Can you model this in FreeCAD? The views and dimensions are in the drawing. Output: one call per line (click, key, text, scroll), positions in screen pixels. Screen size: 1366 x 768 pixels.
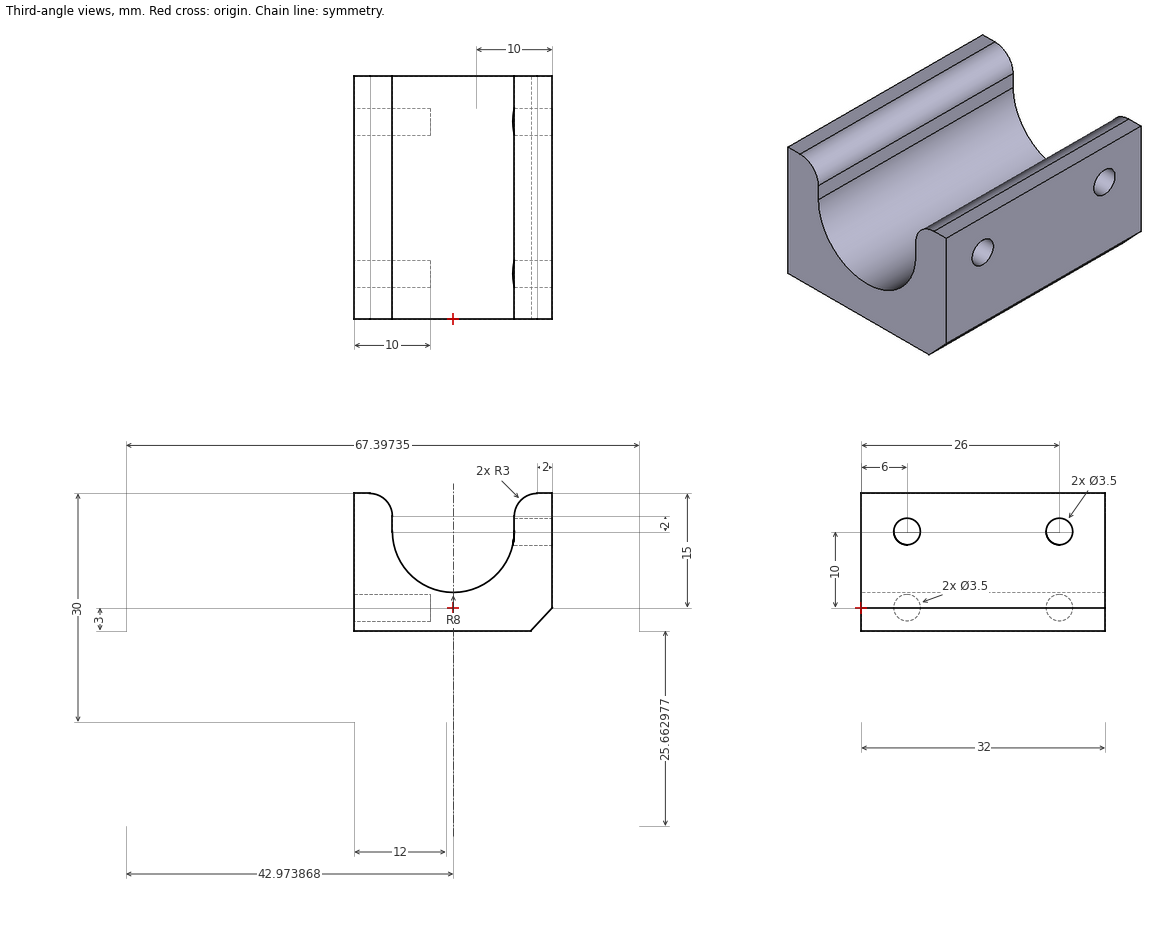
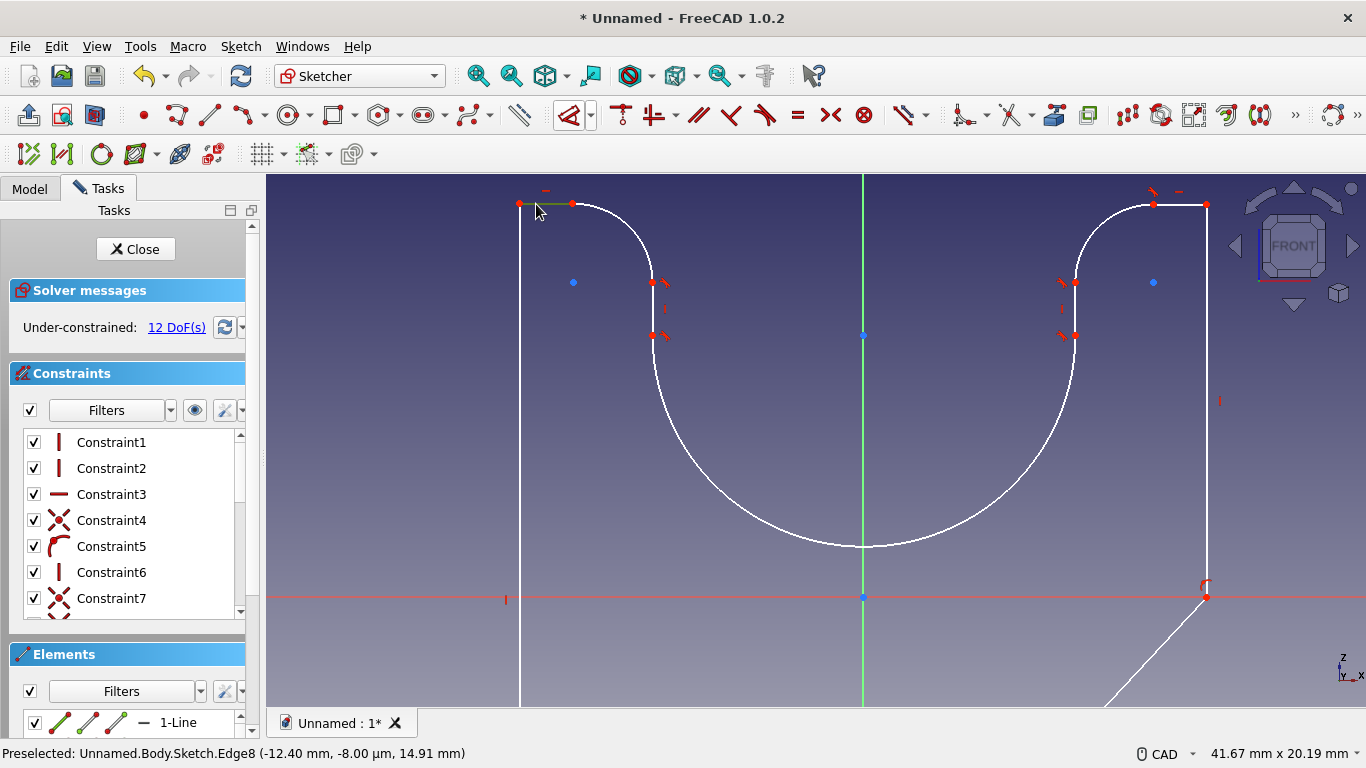
click(644, 246)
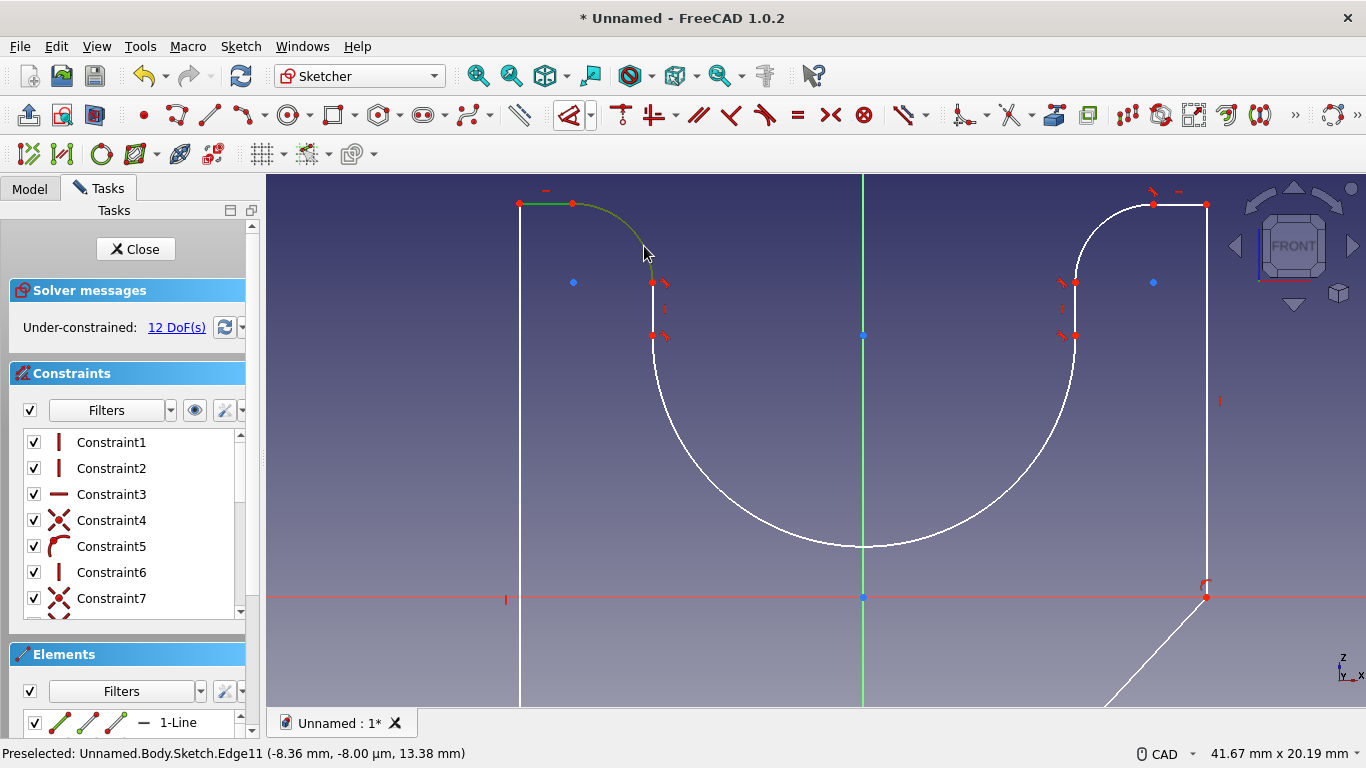
click(765, 116)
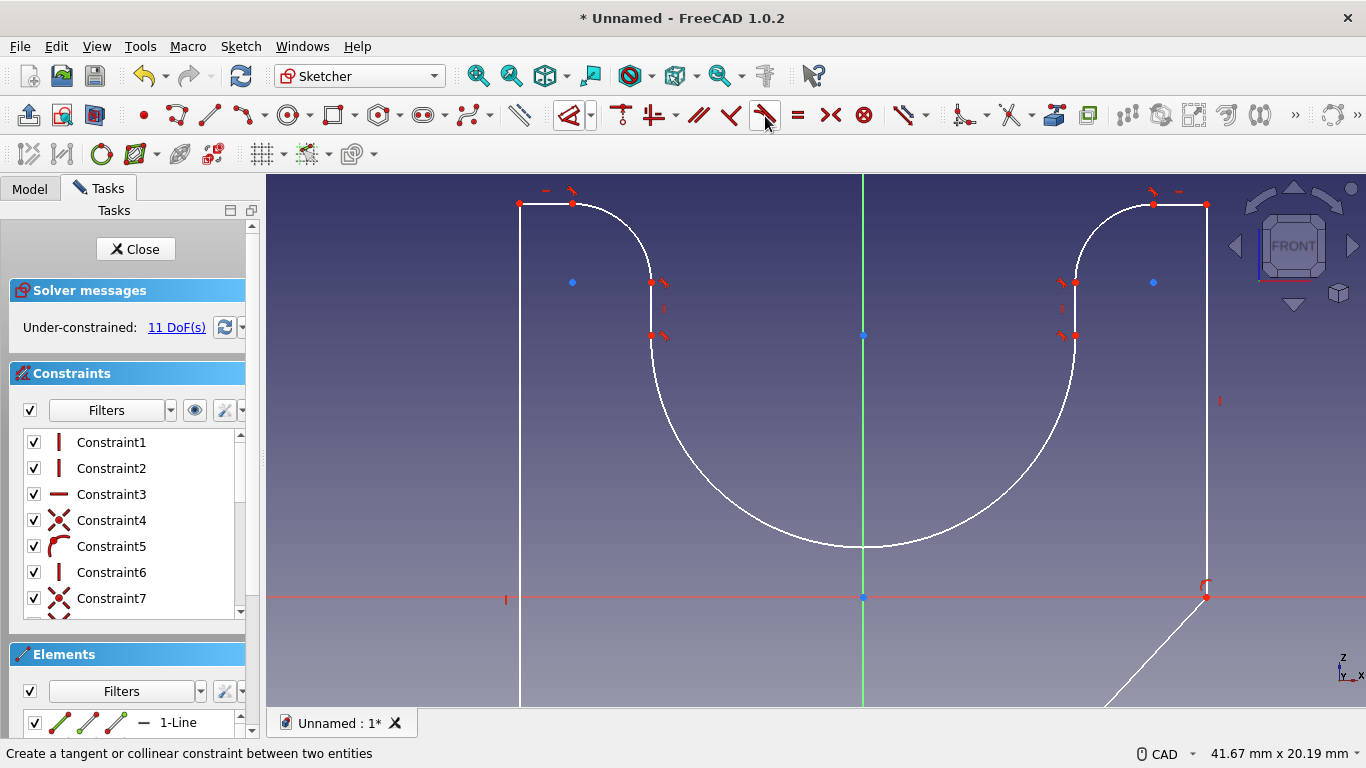
click(1118, 213)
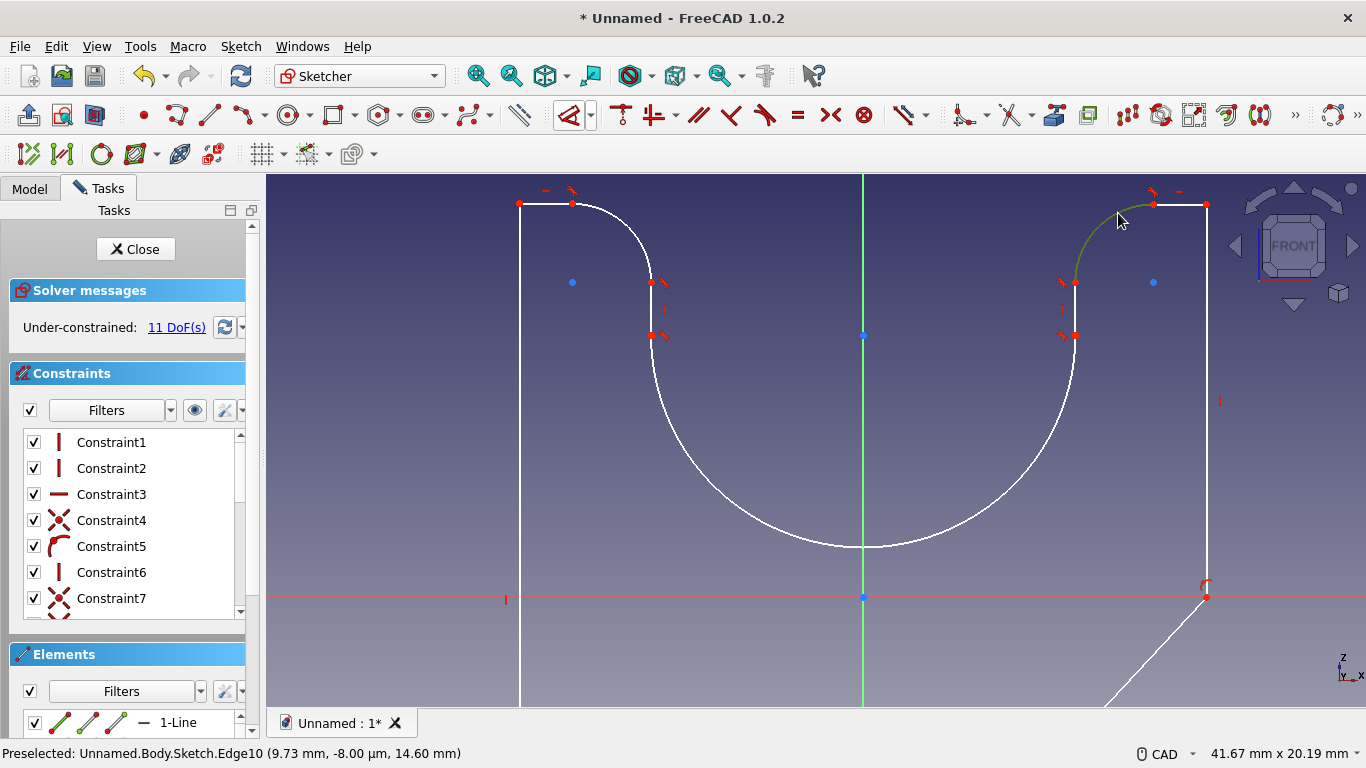
click(642, 247)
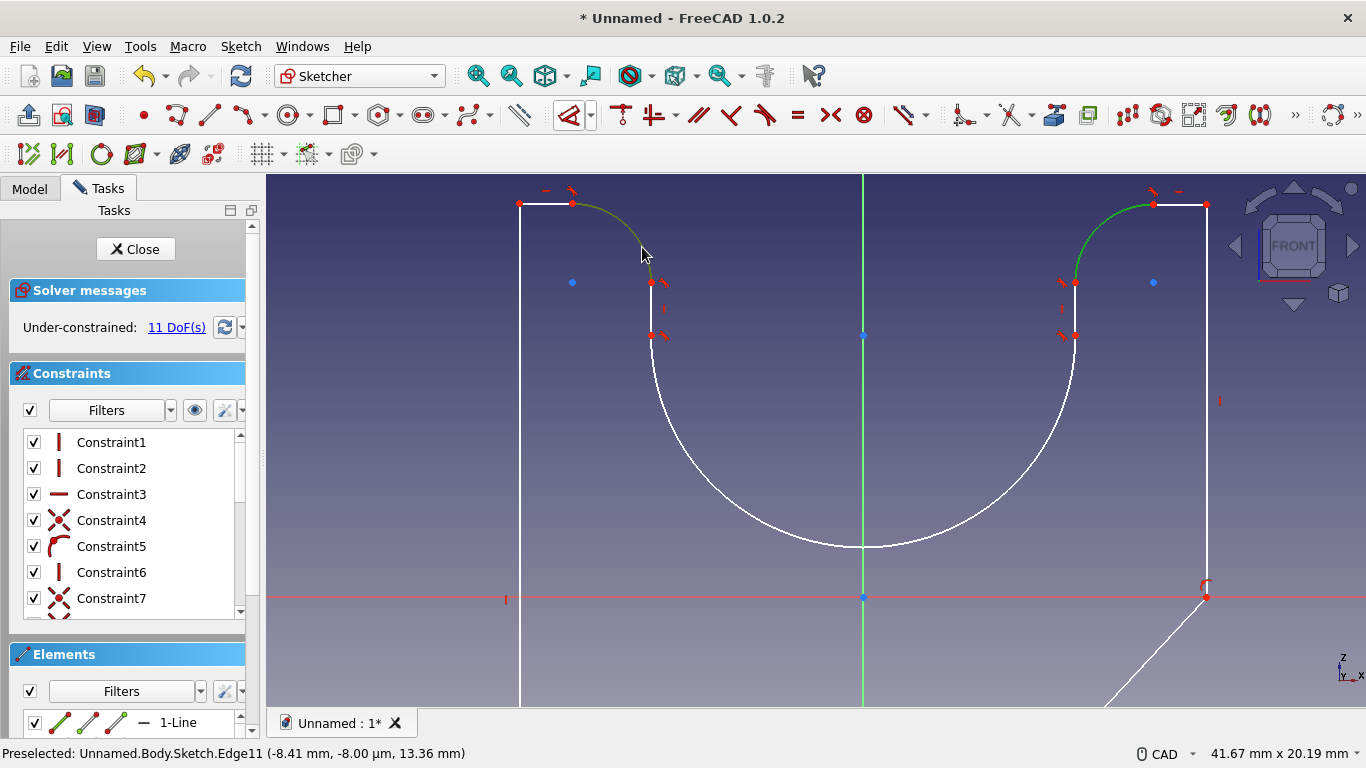
click(798, 116)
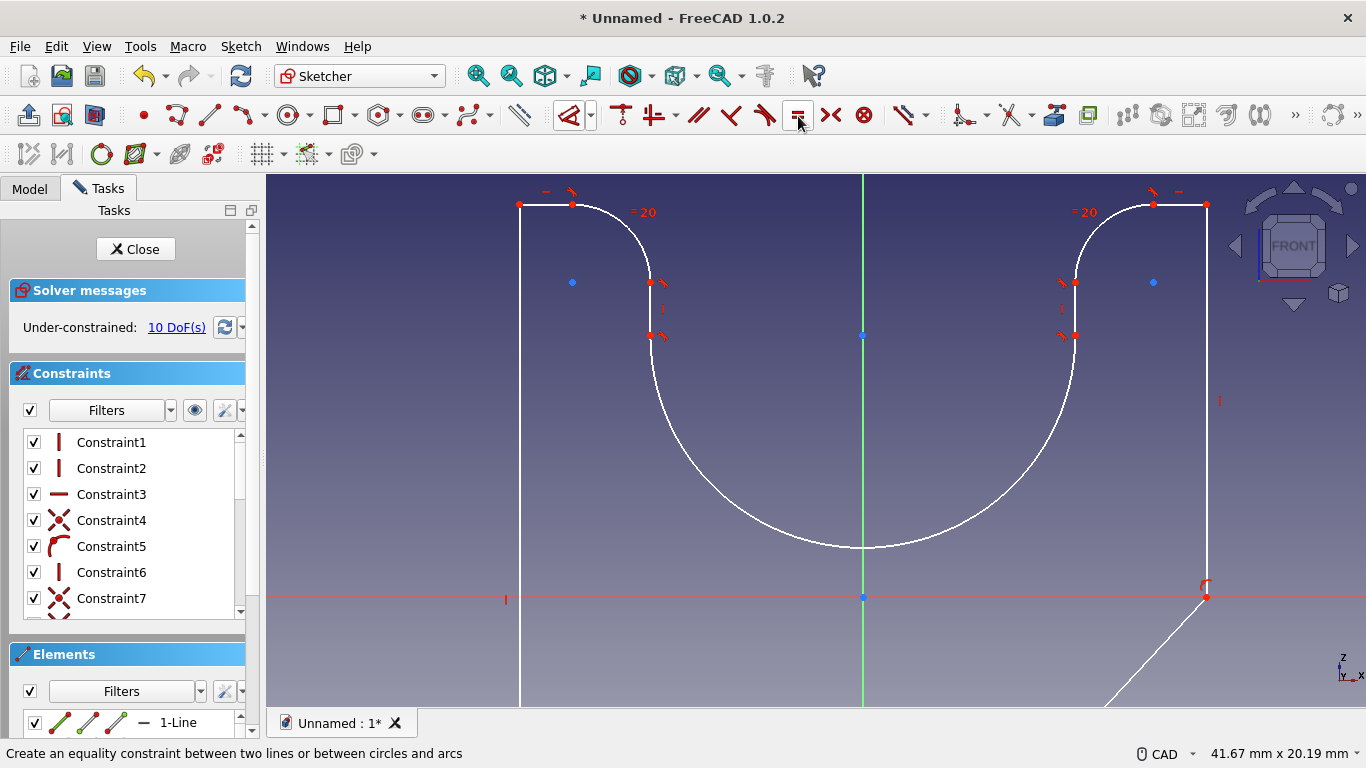
click(863, 335)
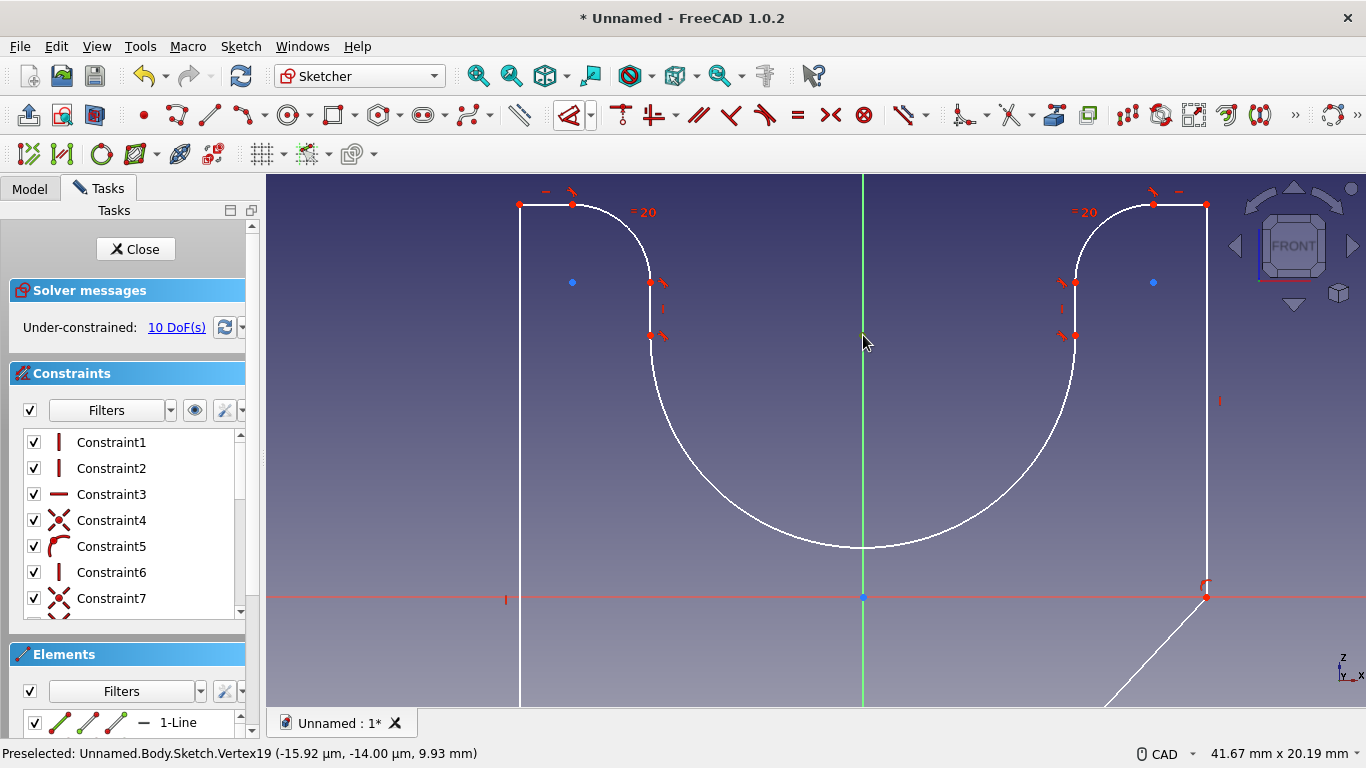
click(863, 645)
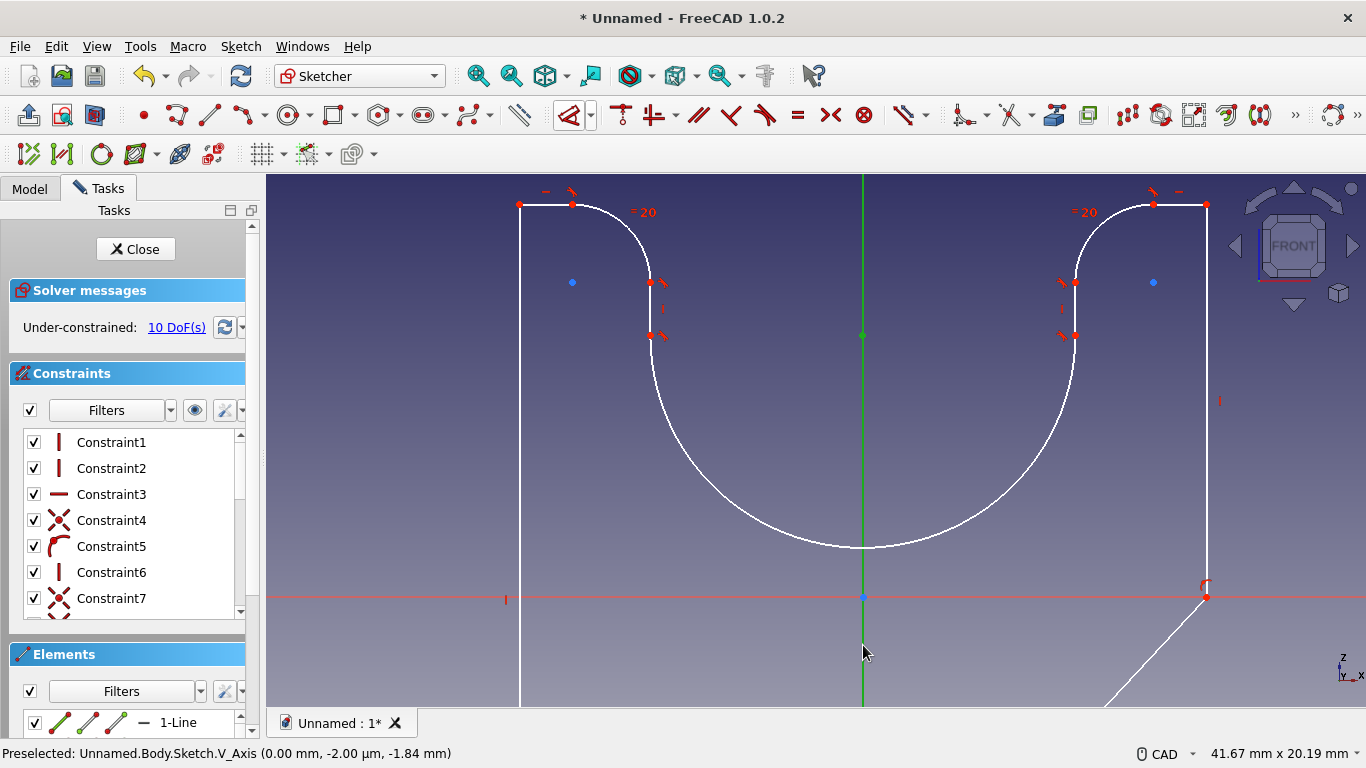
click(621, 116)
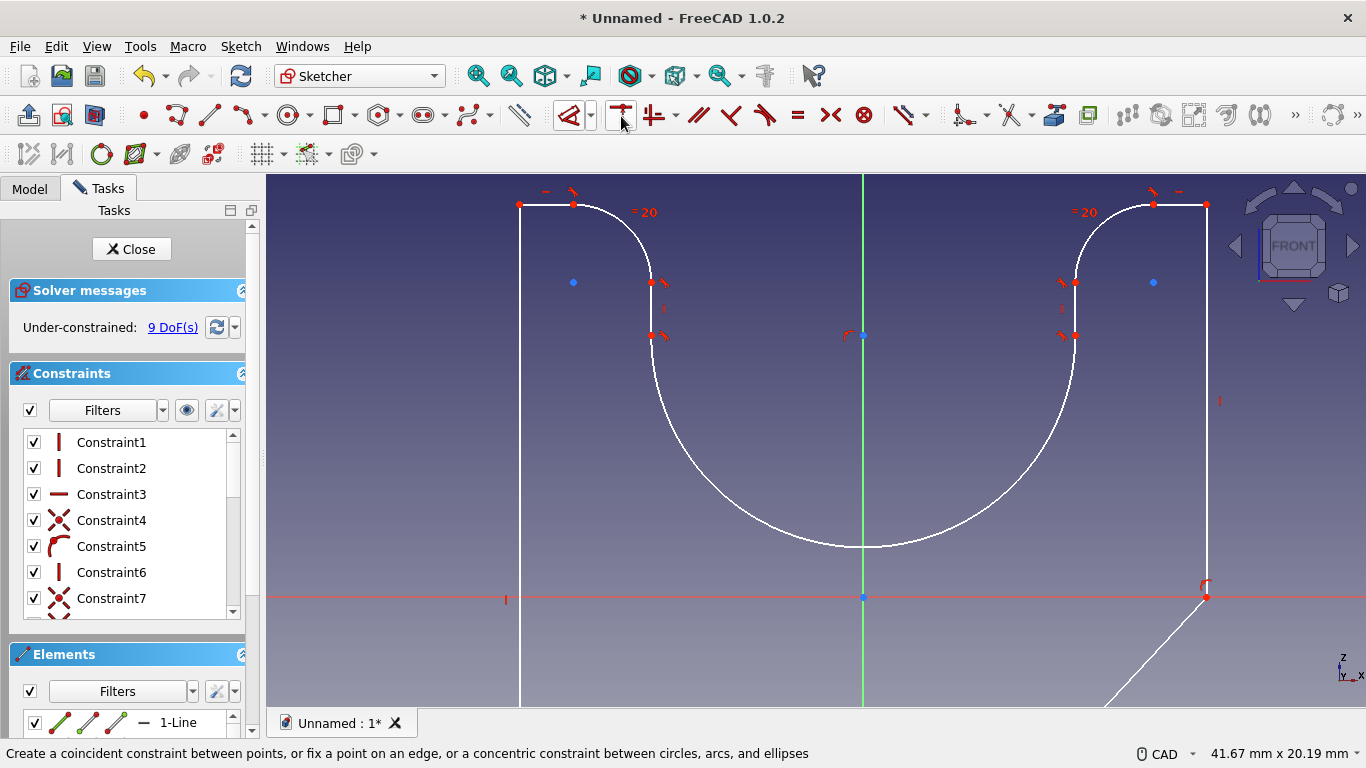
scroll(653, 312, down, 4)